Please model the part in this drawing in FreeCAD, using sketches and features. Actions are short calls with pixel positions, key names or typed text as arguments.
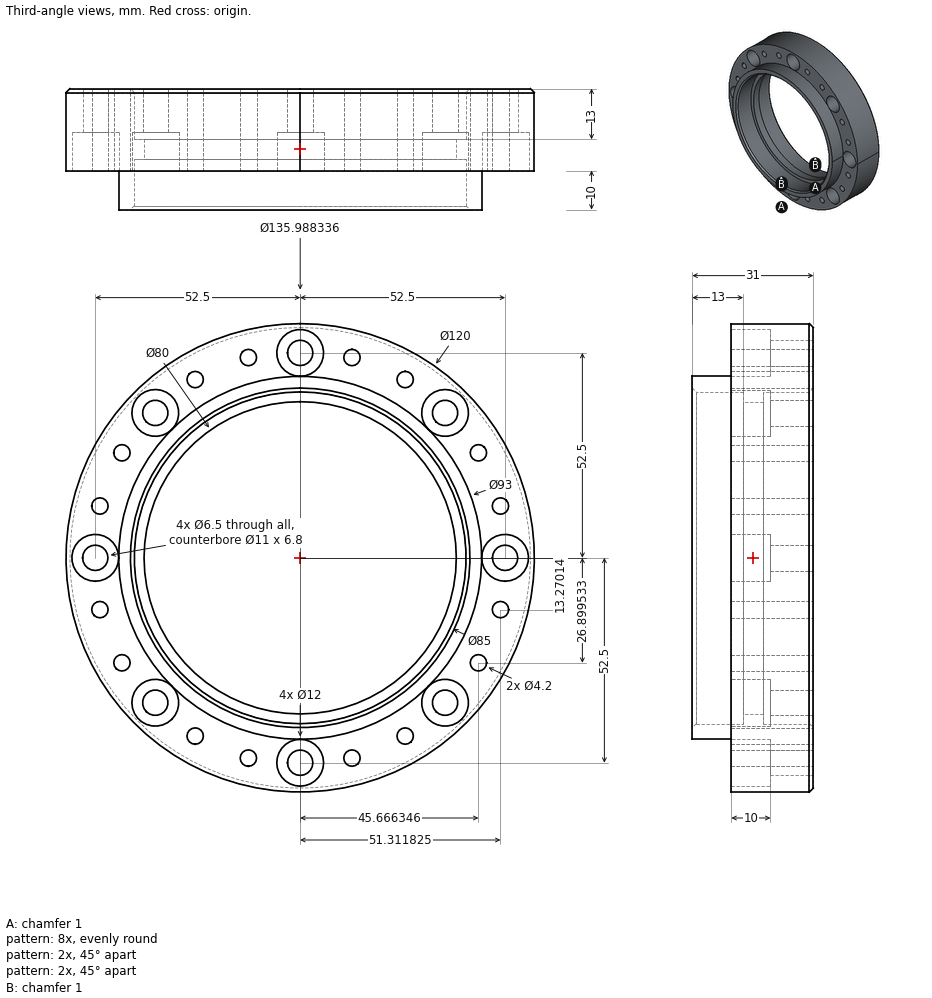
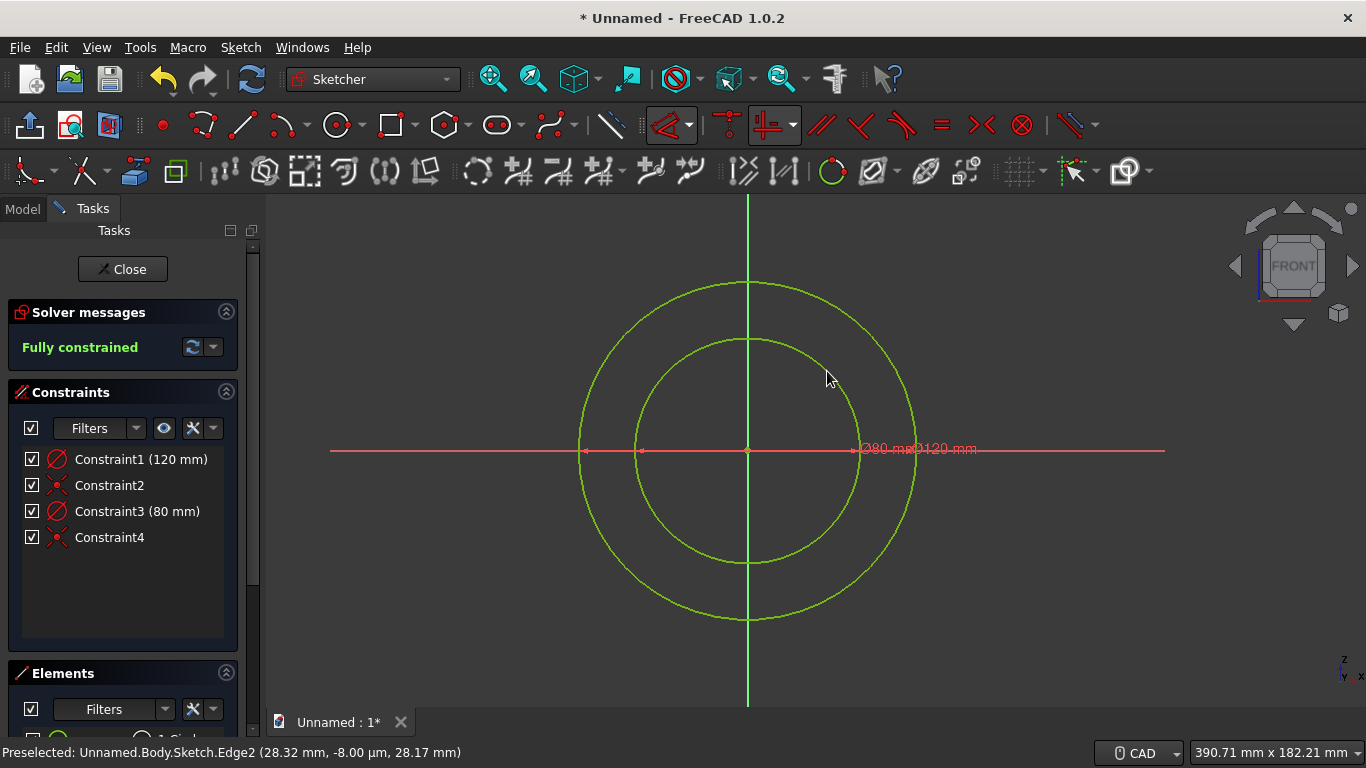
click(123, 269)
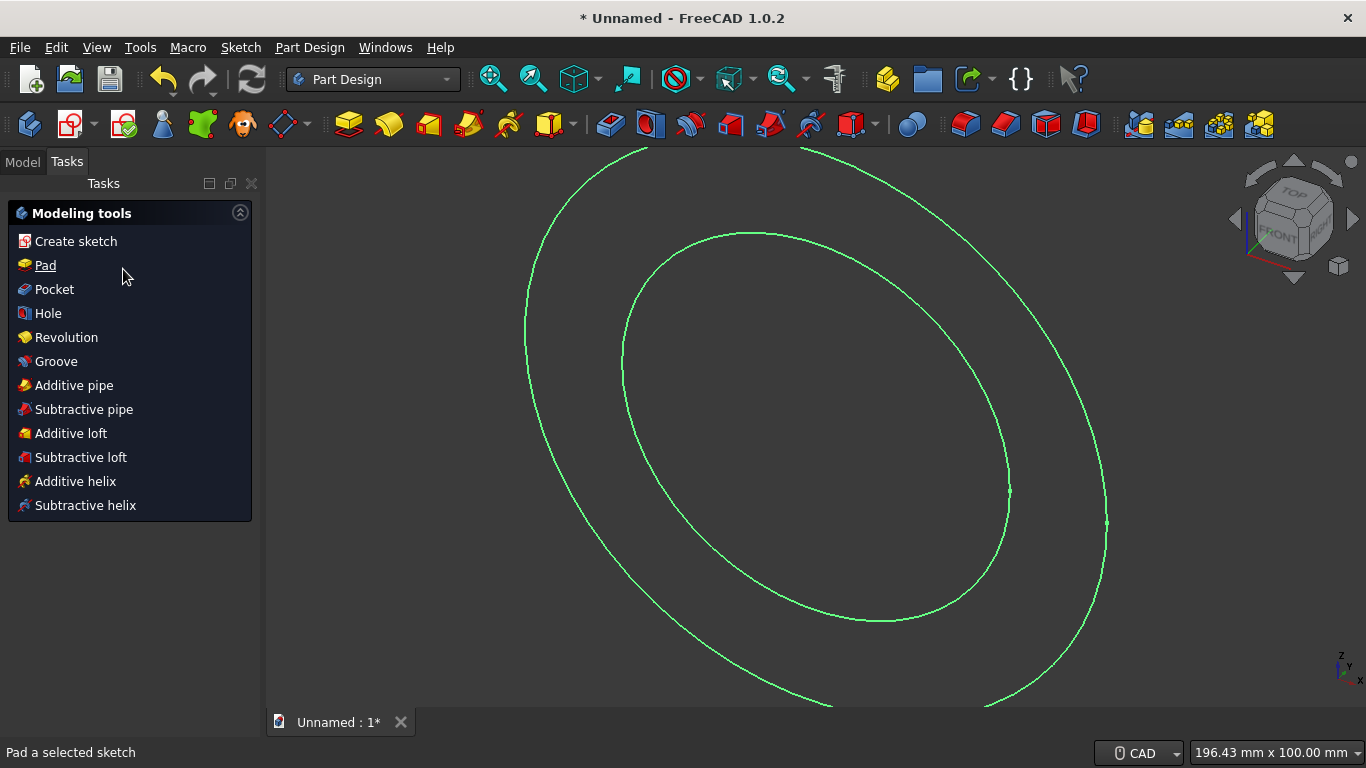
click(350, 124)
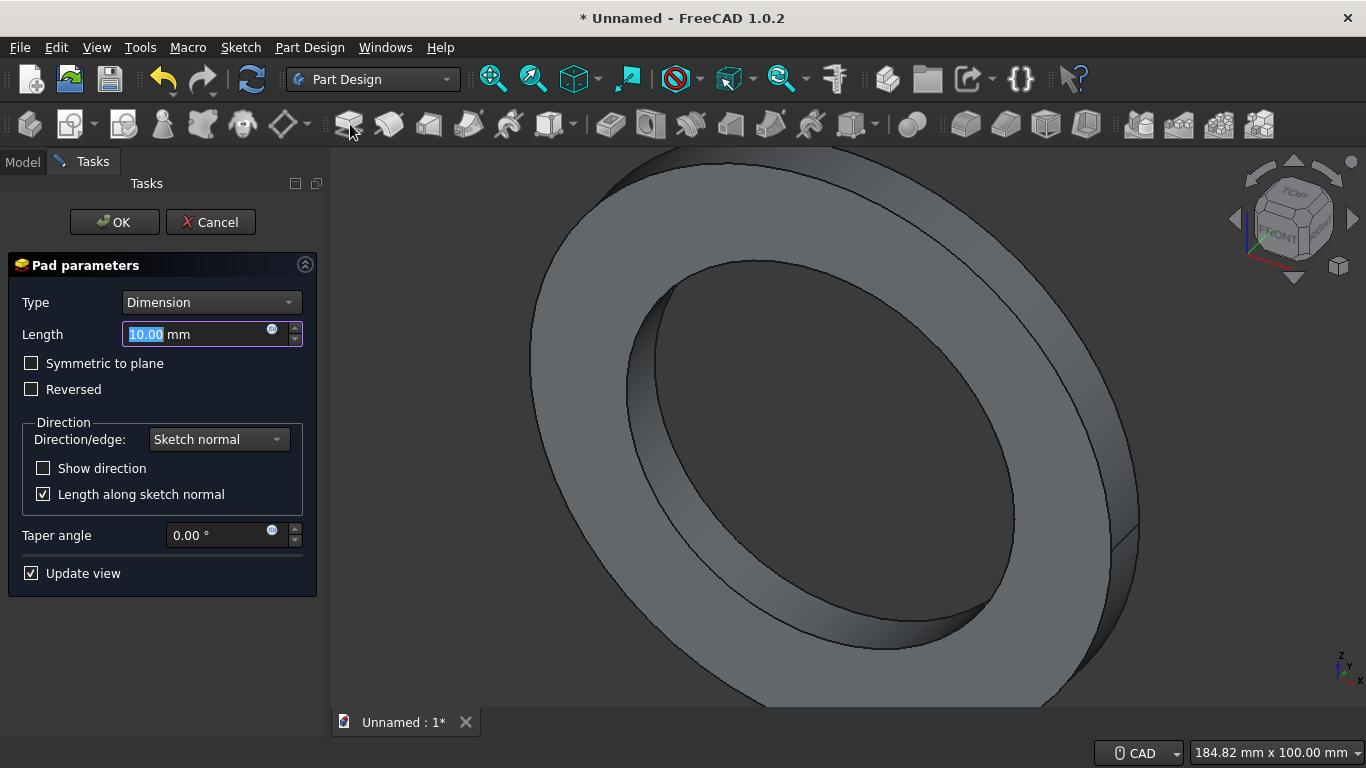
text(31)
key(Tab)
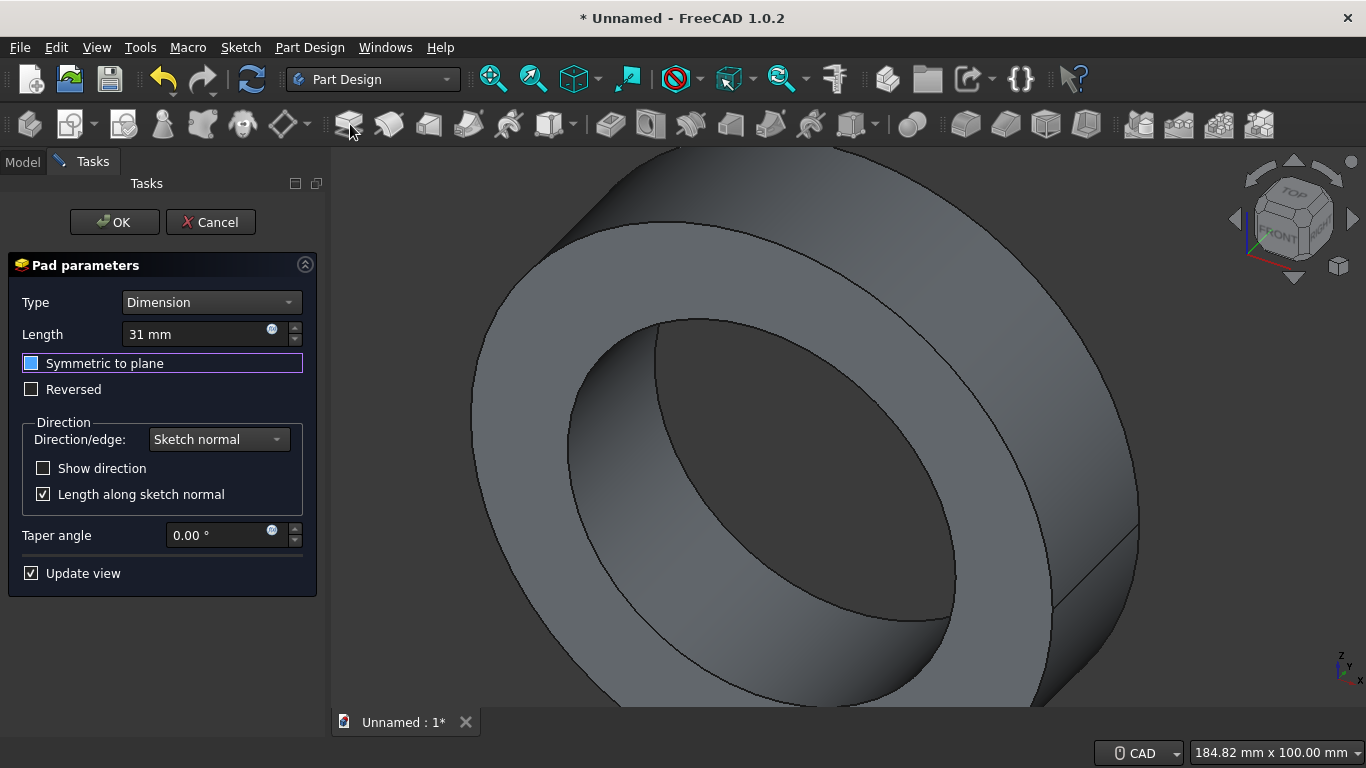
click(30, 363)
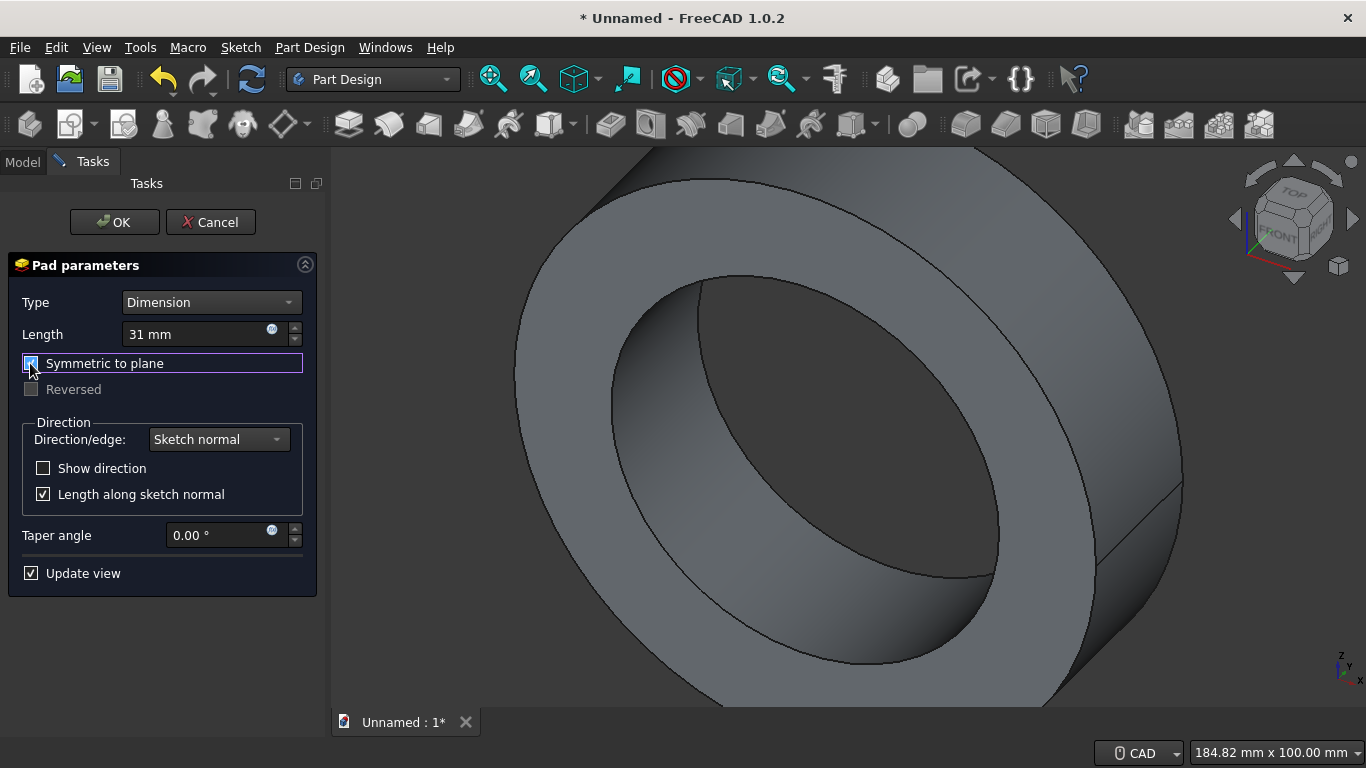
click(115, 222)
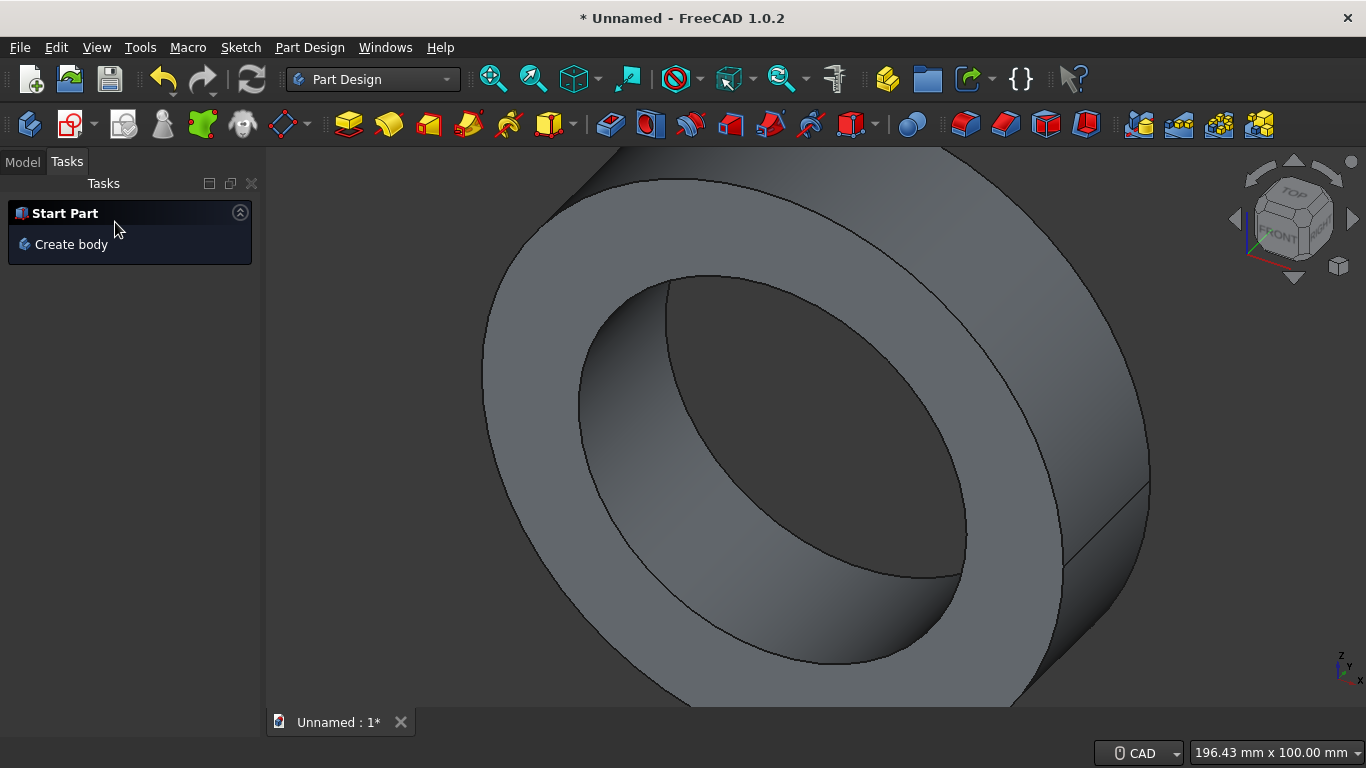
click(494, 80)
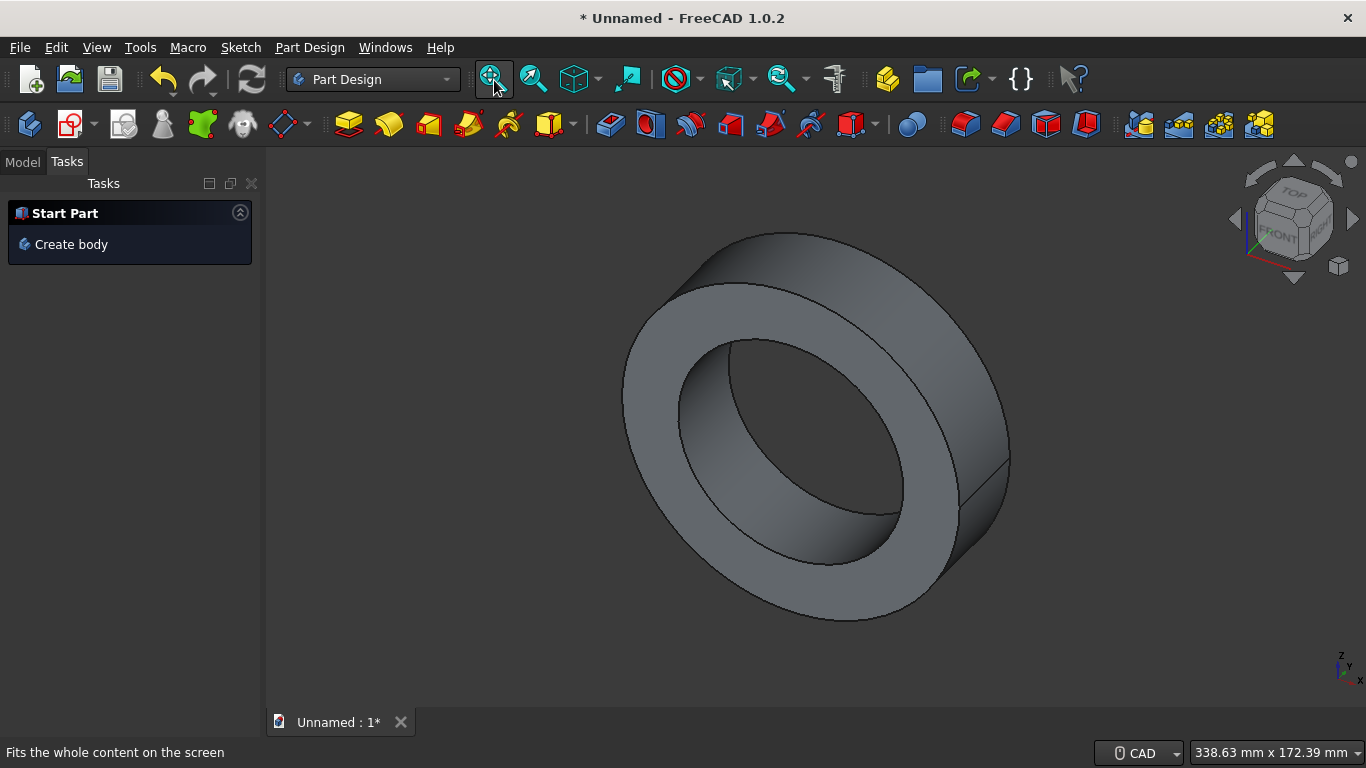
click(654, 312)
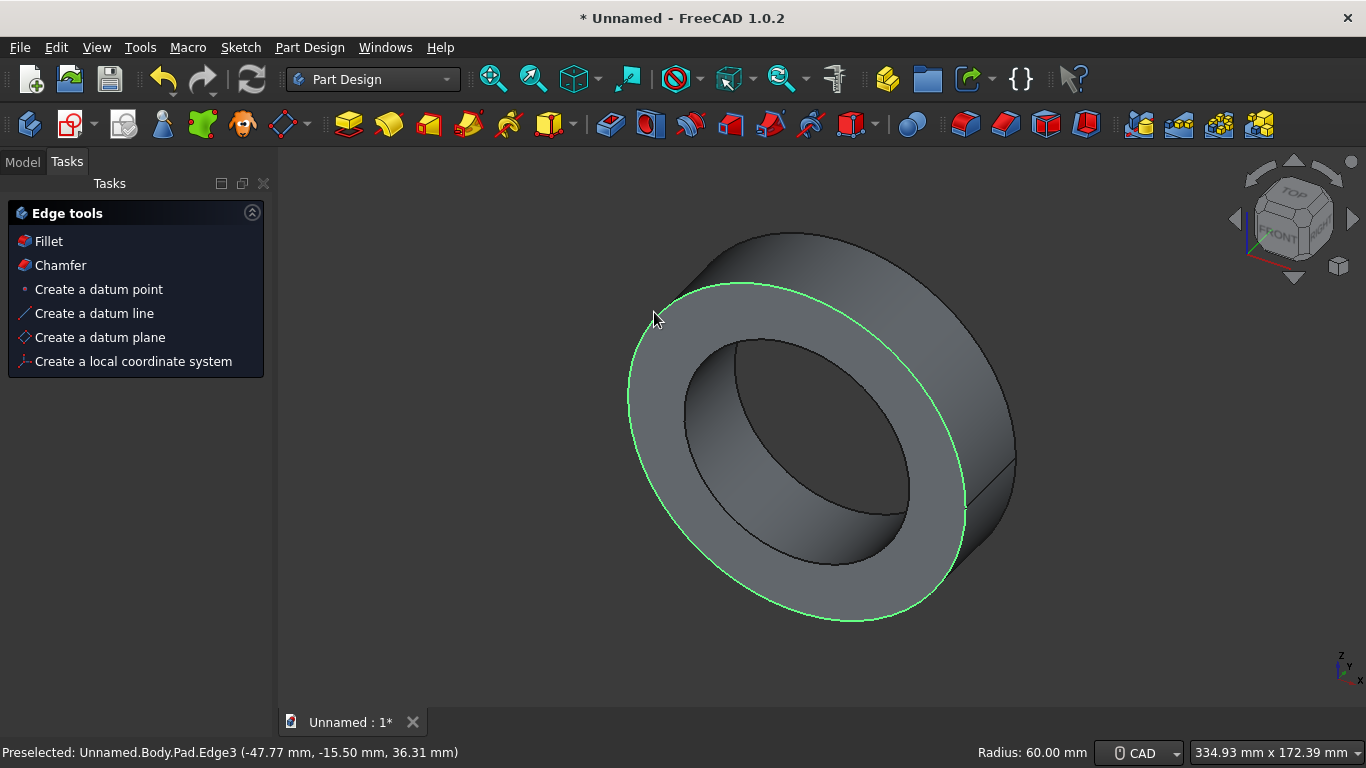
click(684, 414, ctrl)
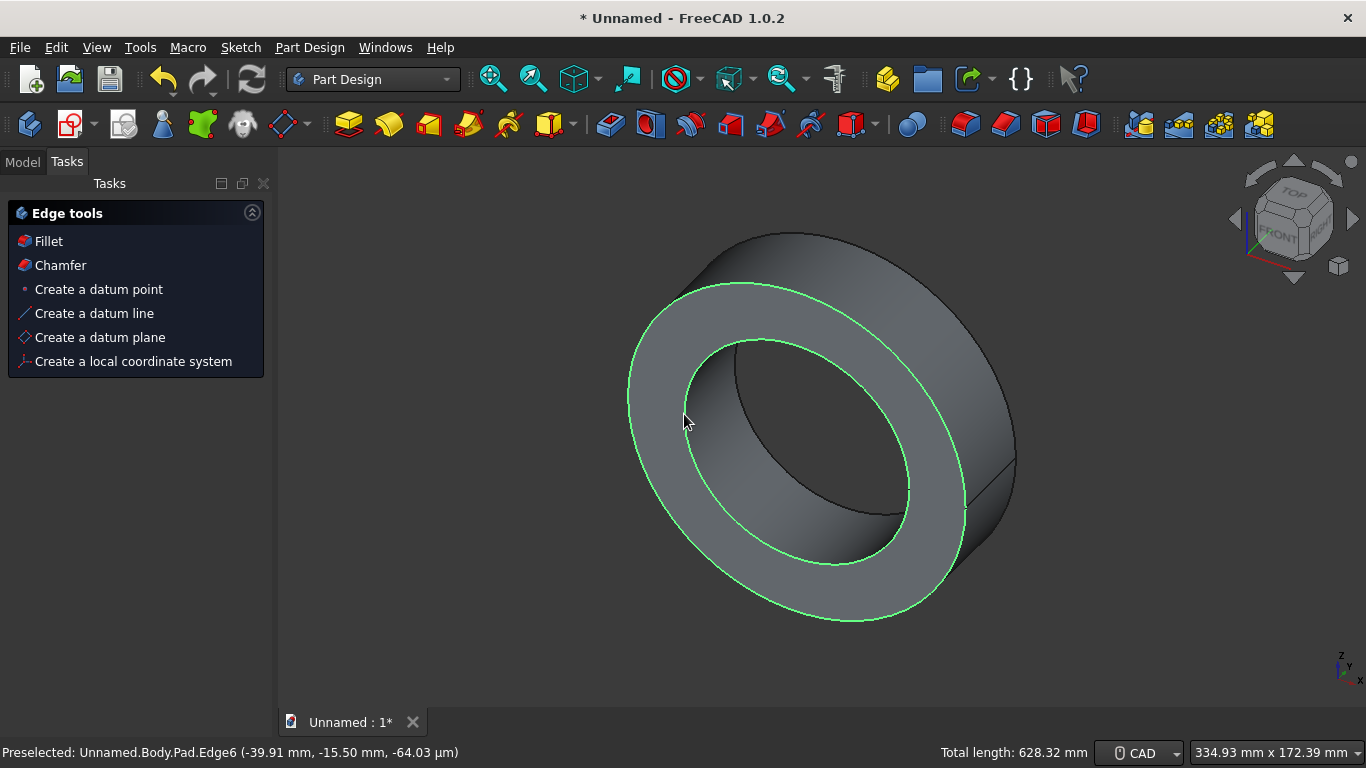
key(0)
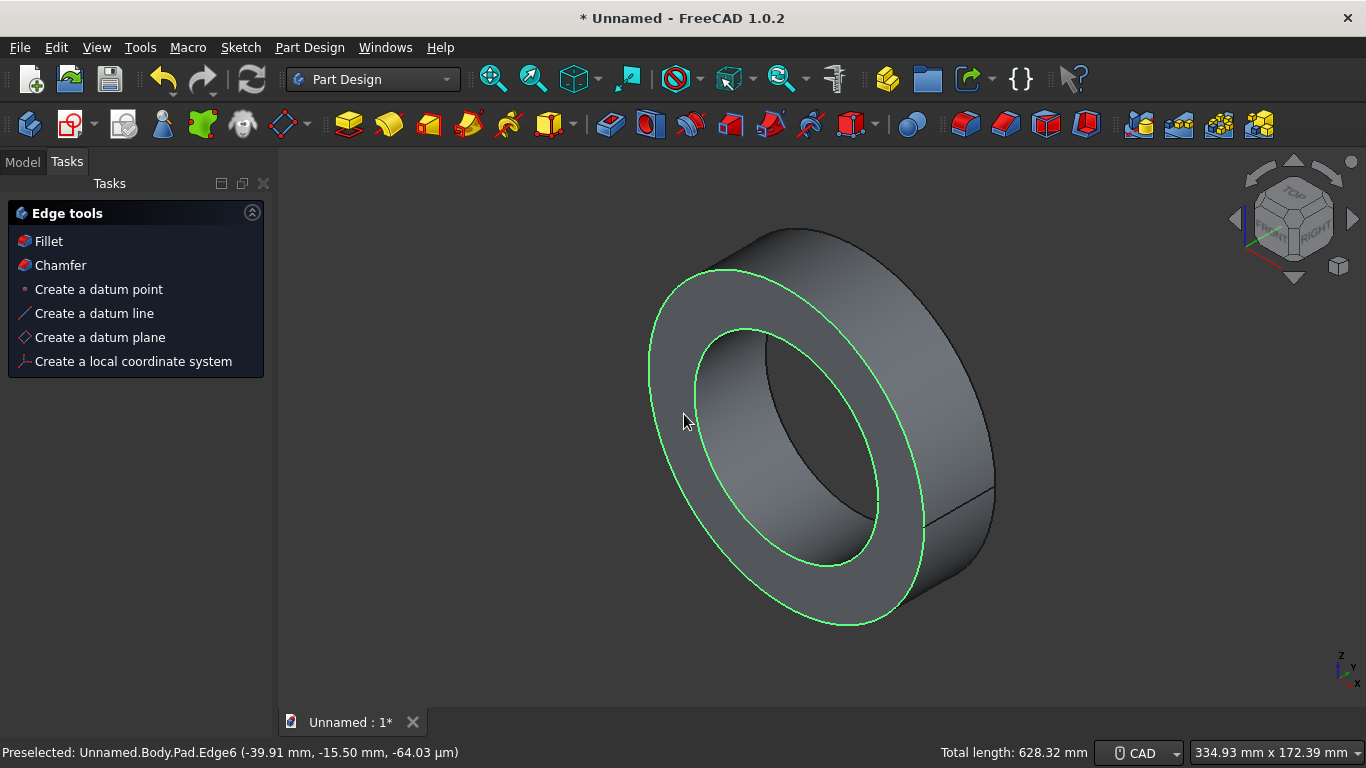
key(2)